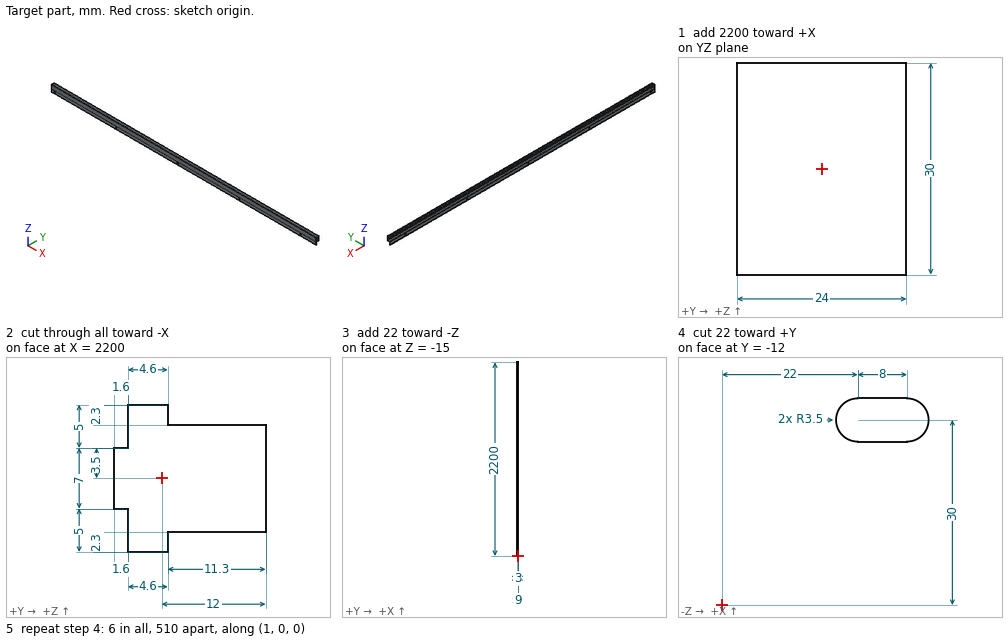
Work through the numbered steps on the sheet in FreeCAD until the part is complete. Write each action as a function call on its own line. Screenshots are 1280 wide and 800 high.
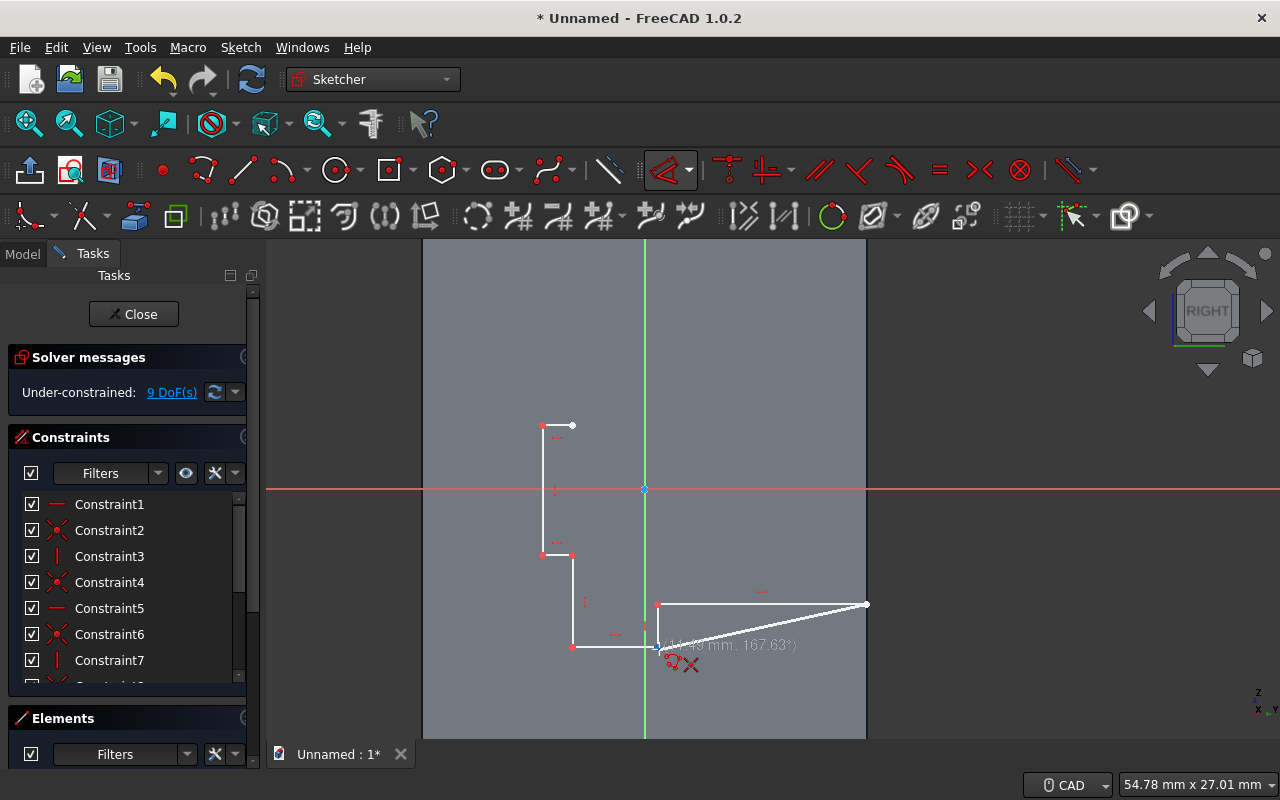
click(867, 374)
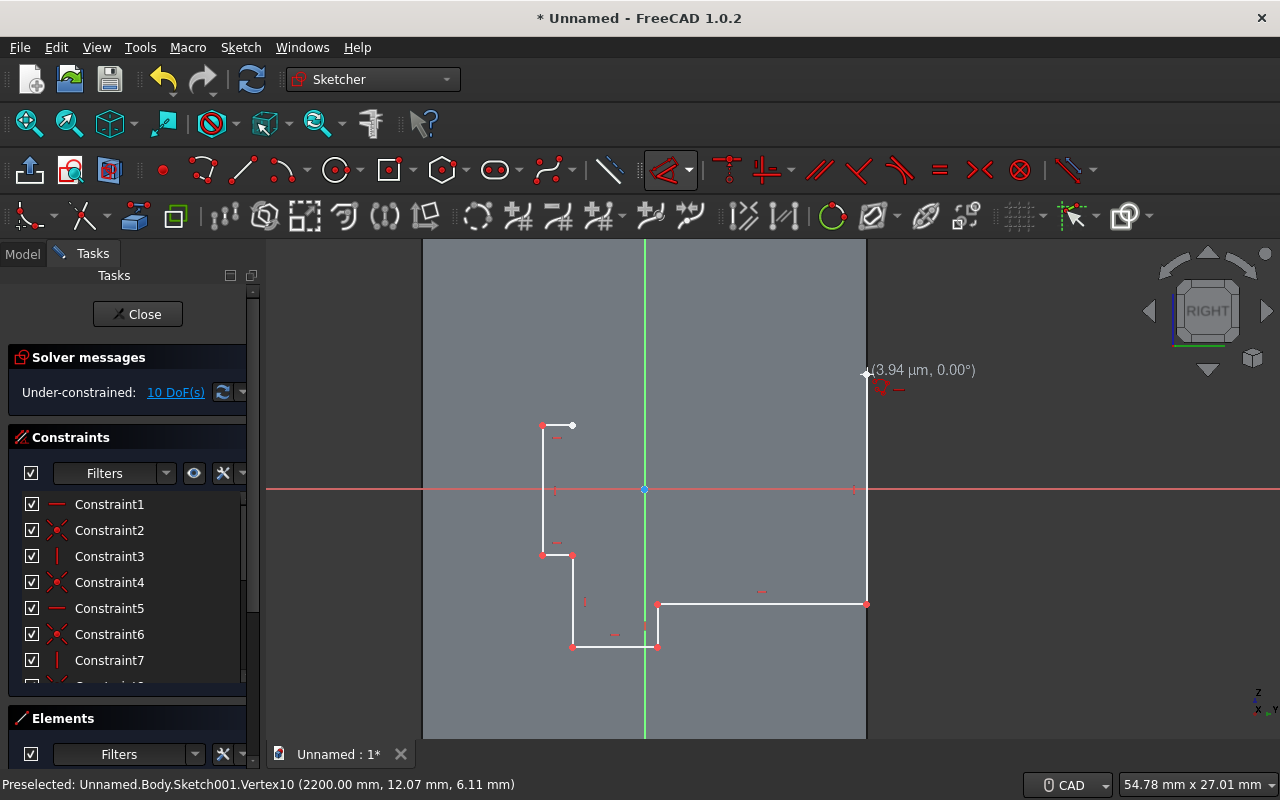
scroll(658, 374, up, 2)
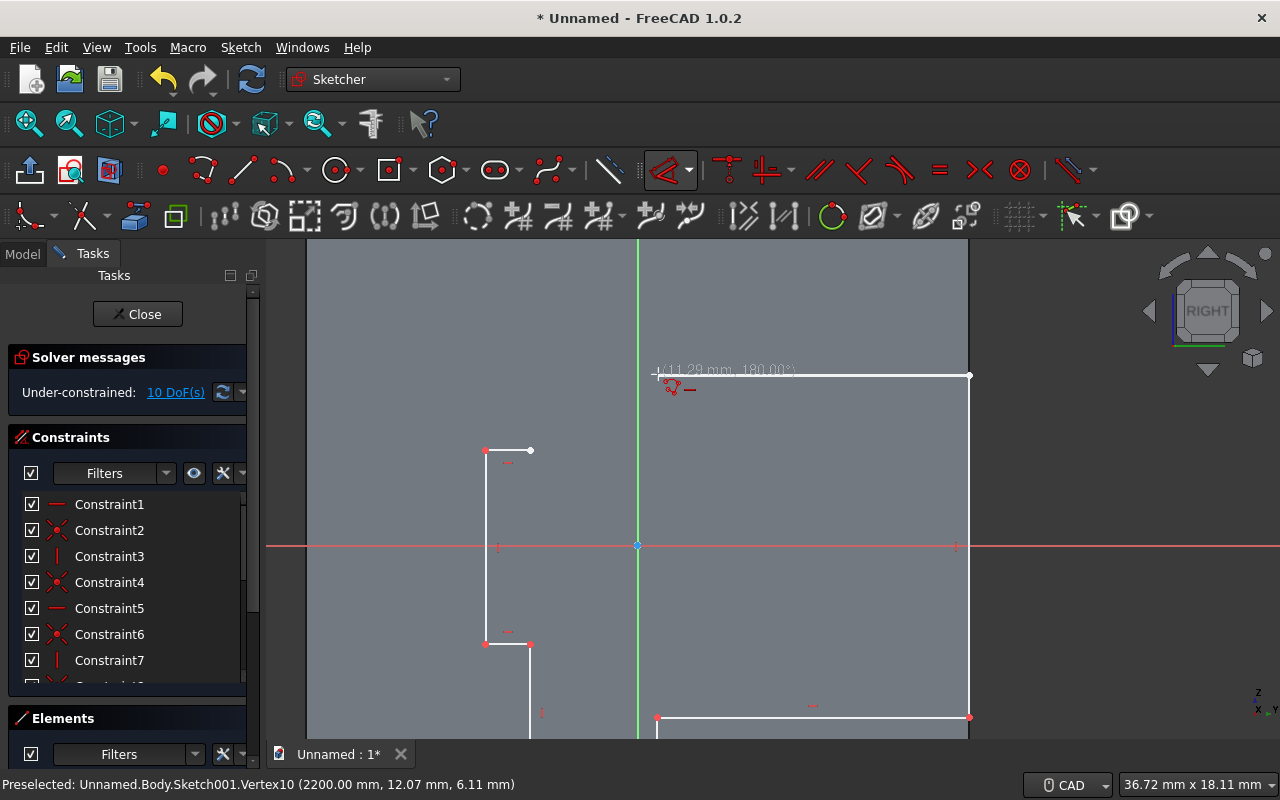
click(657, 374)
click(657, 311)
click(530, 311)
click(530, 450)
key(Escape)
key(Escape)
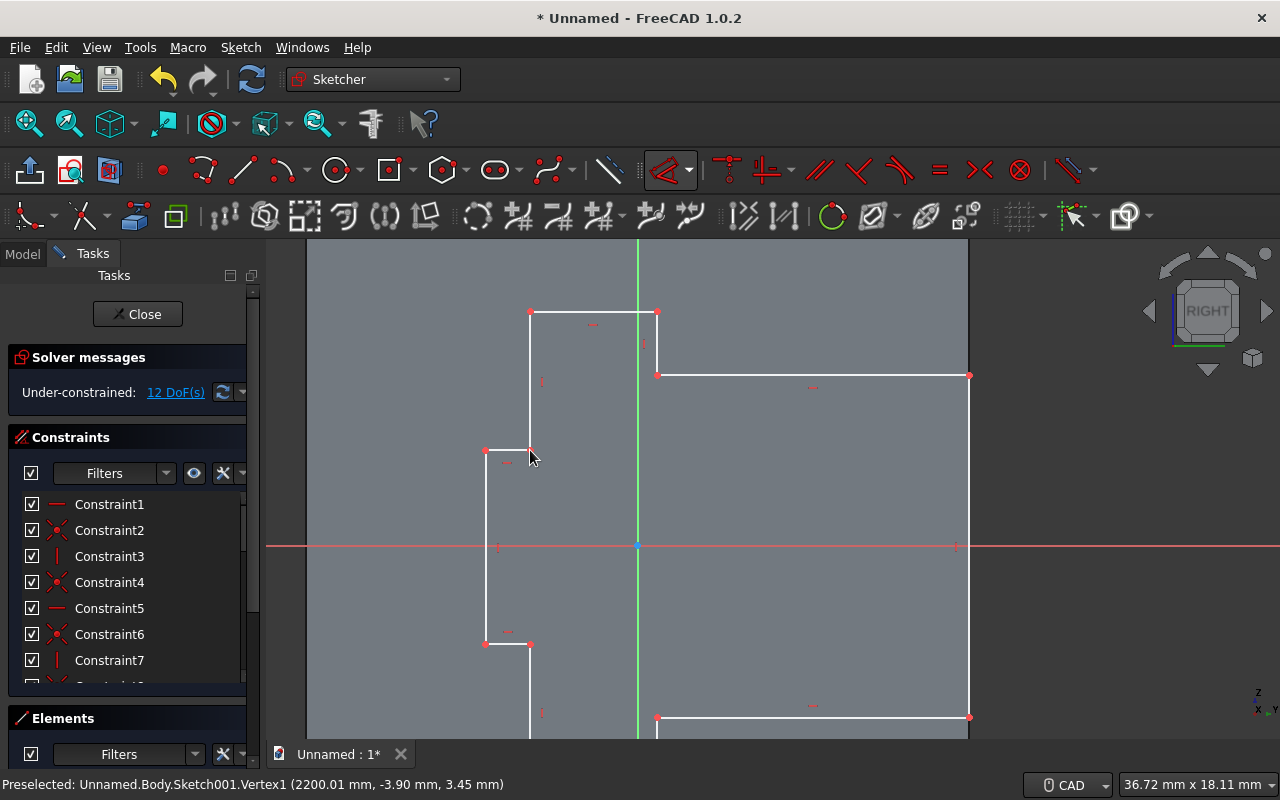
click(486, 509)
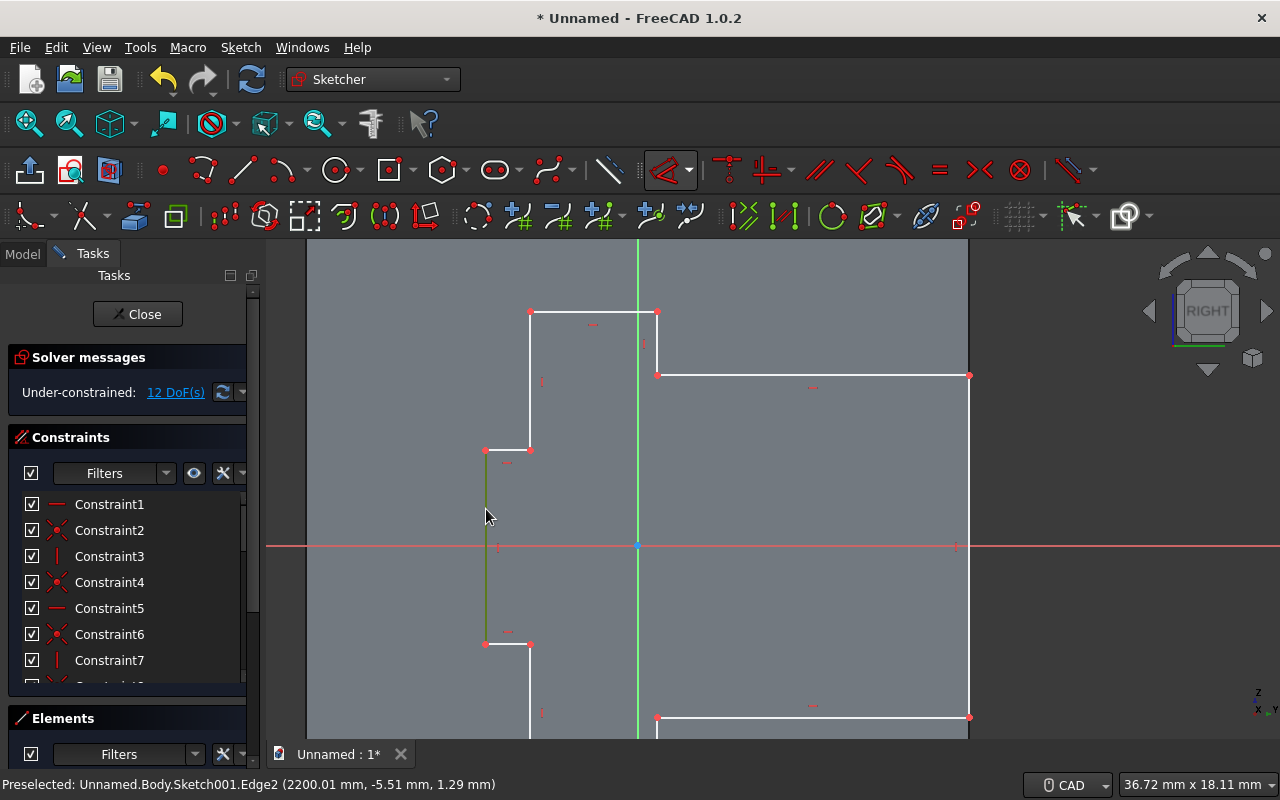
key(i)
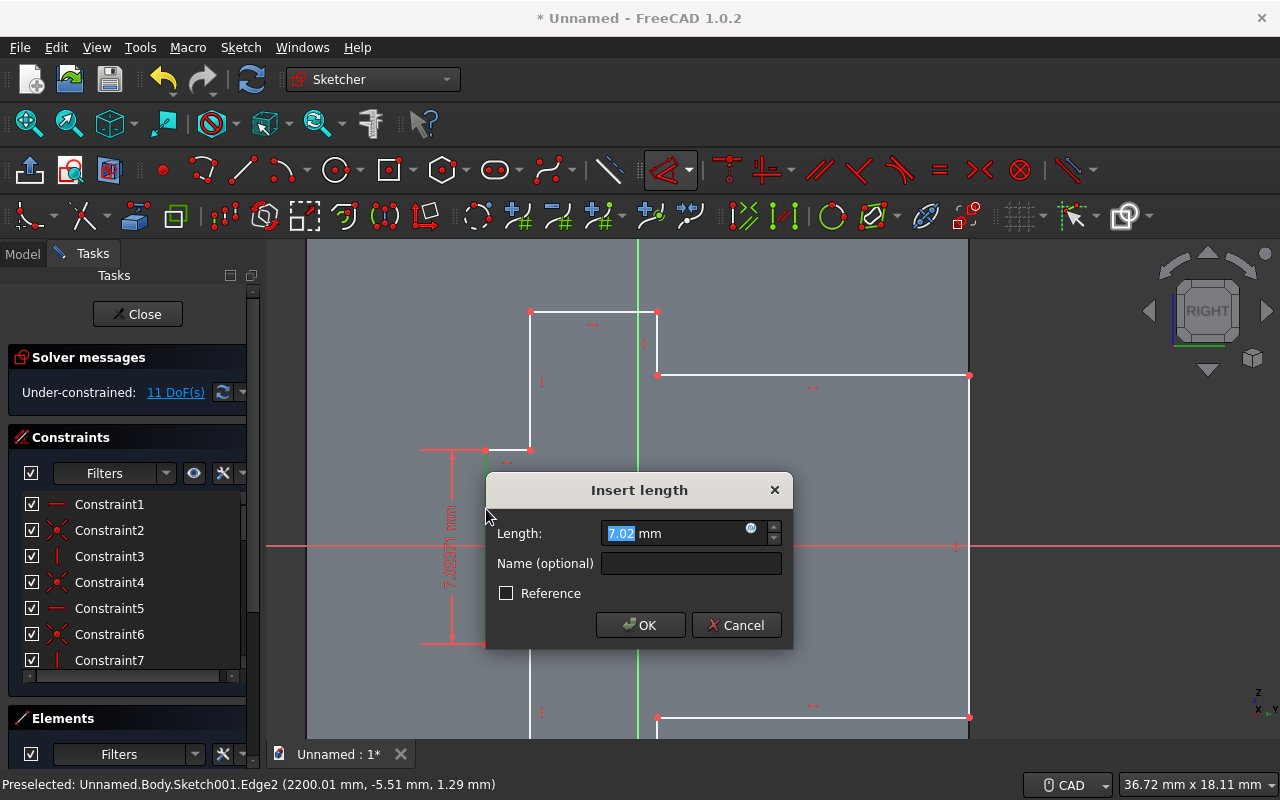
text(7)
key(Return)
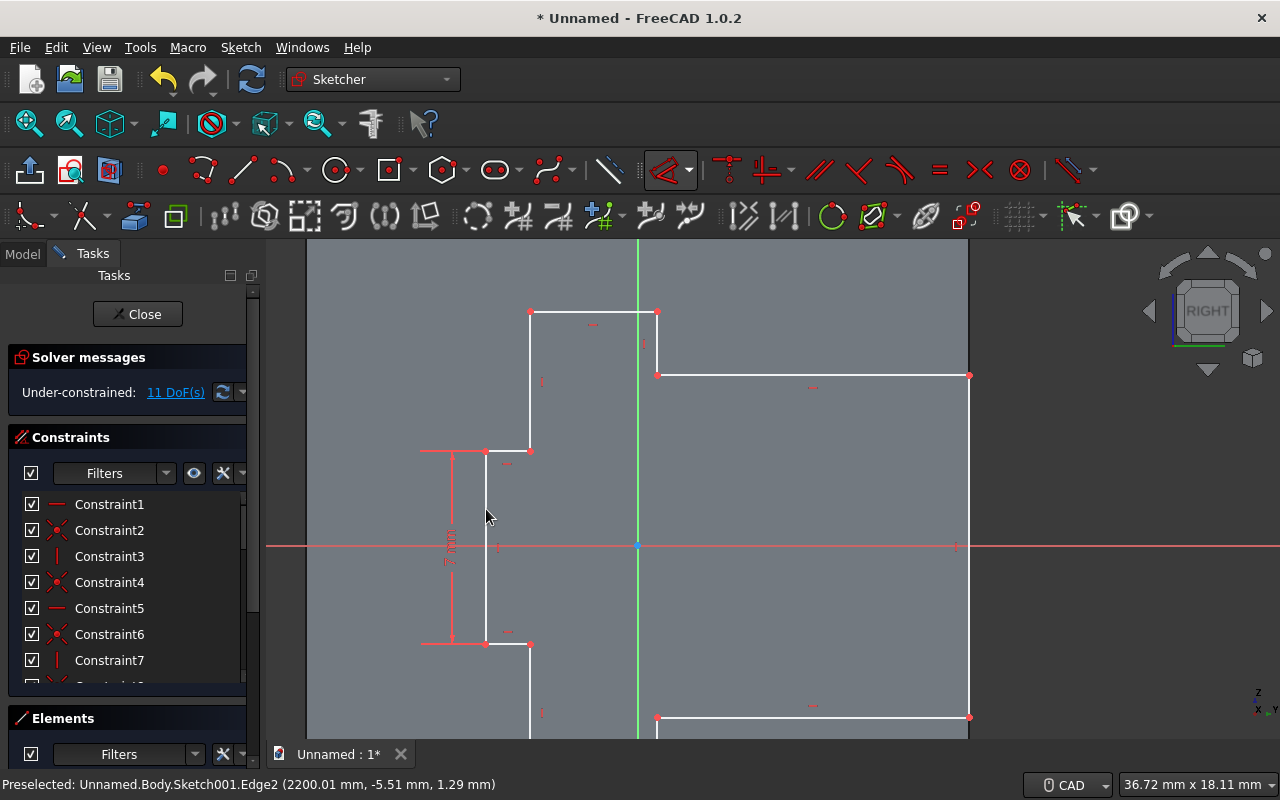
click(530, 686)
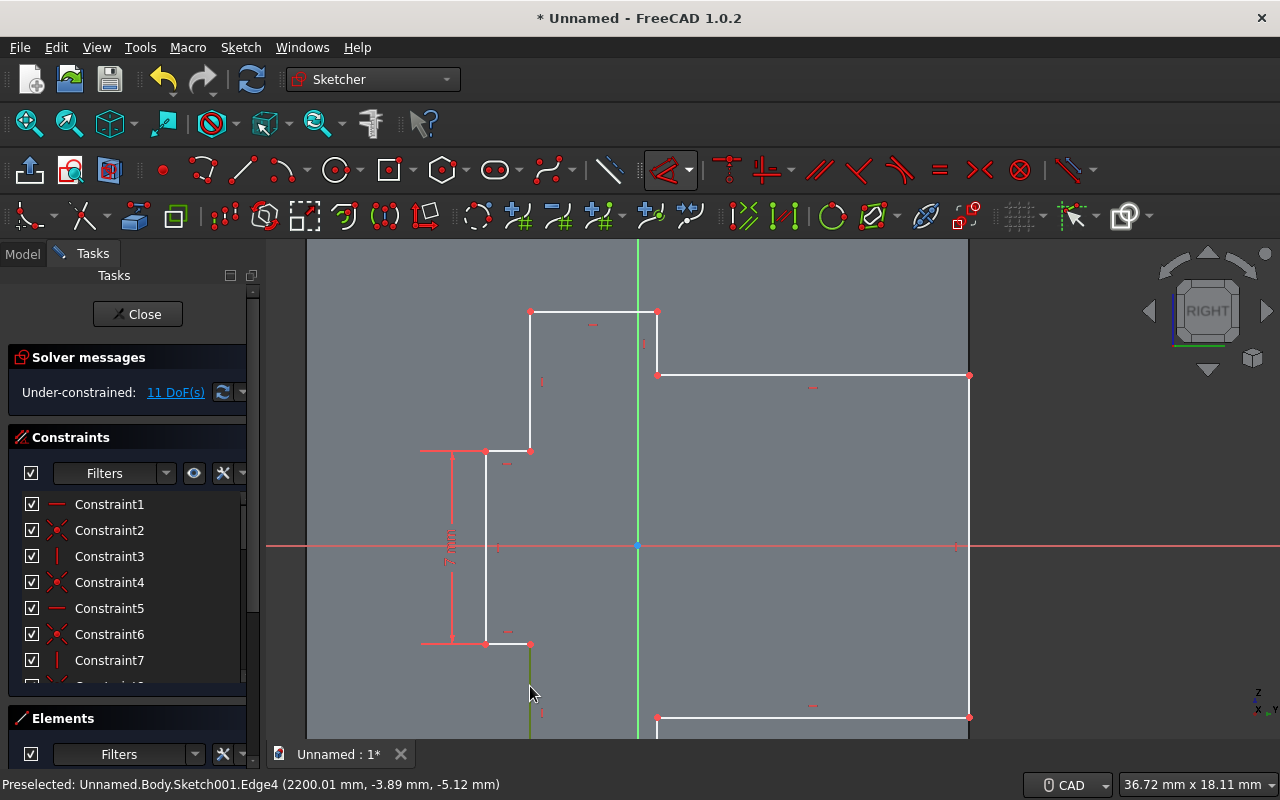
click(692, 170)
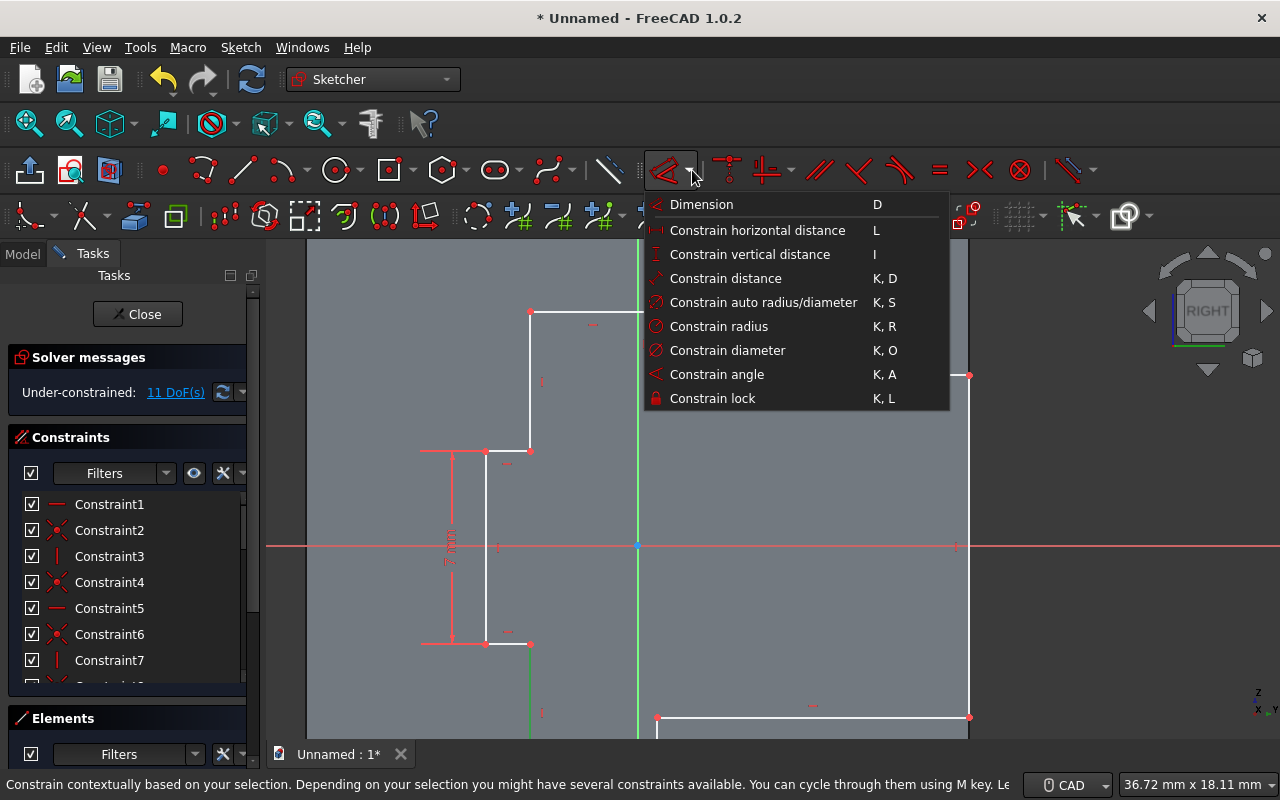
click(797, 254)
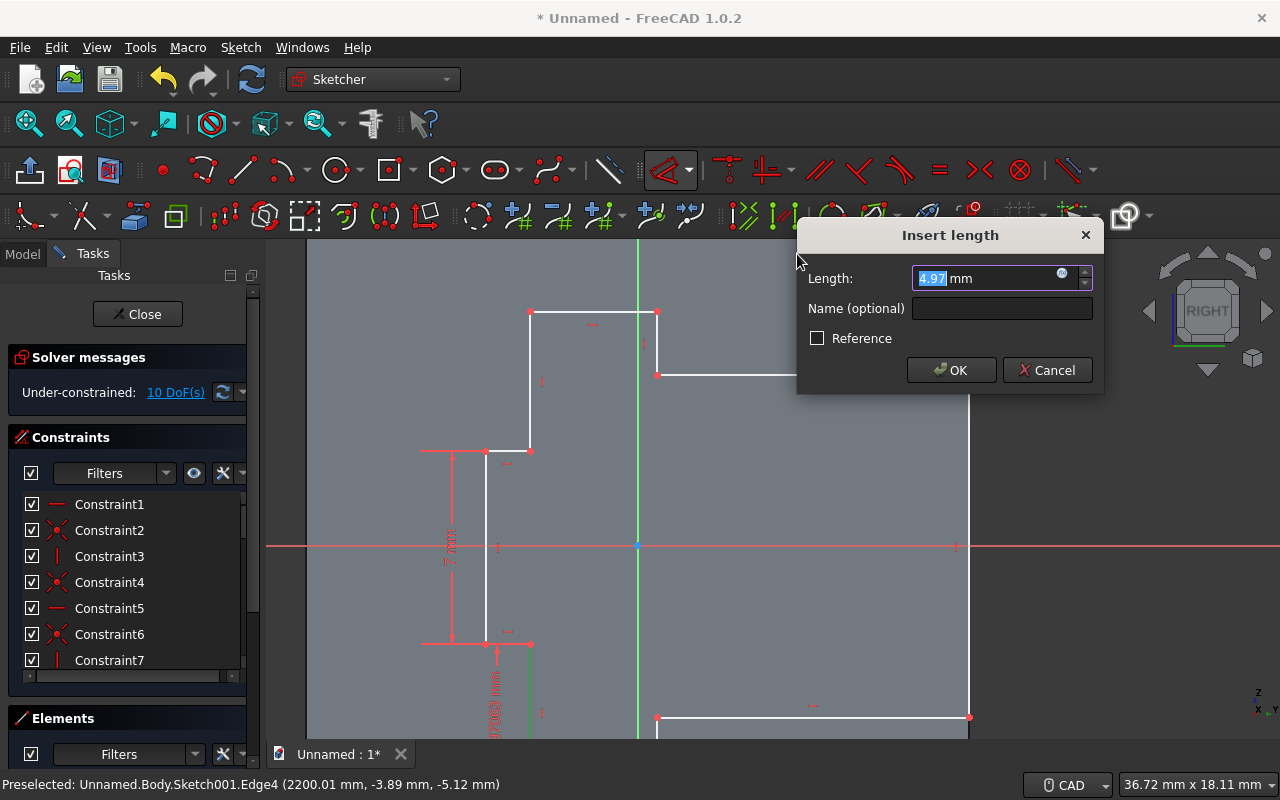
text(5)
key(Return)